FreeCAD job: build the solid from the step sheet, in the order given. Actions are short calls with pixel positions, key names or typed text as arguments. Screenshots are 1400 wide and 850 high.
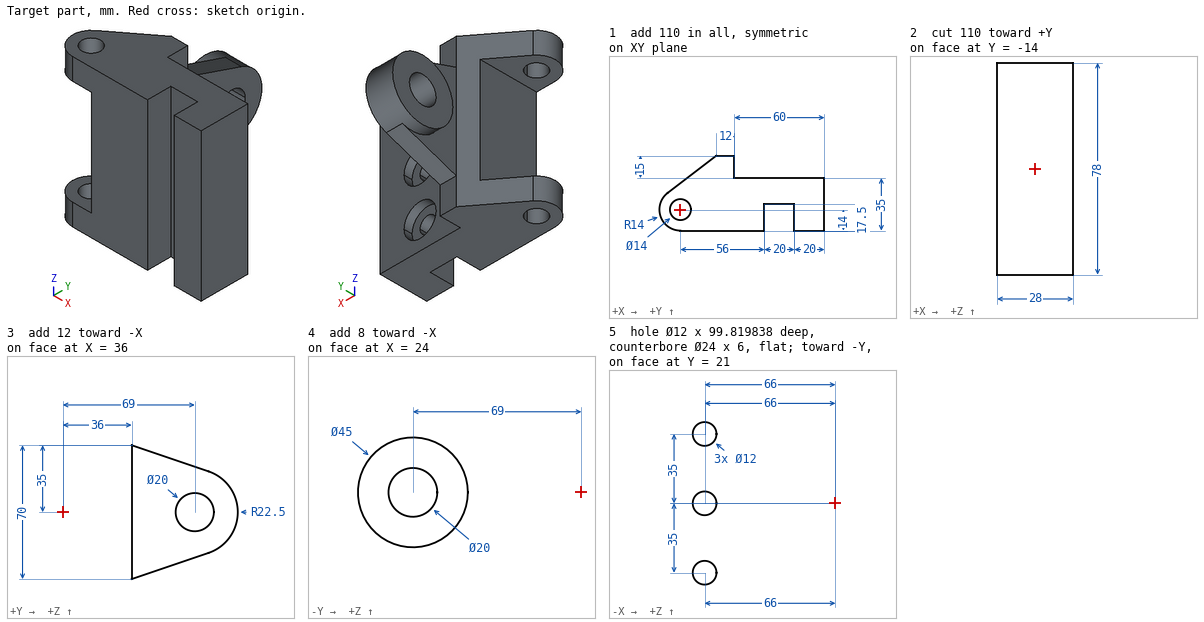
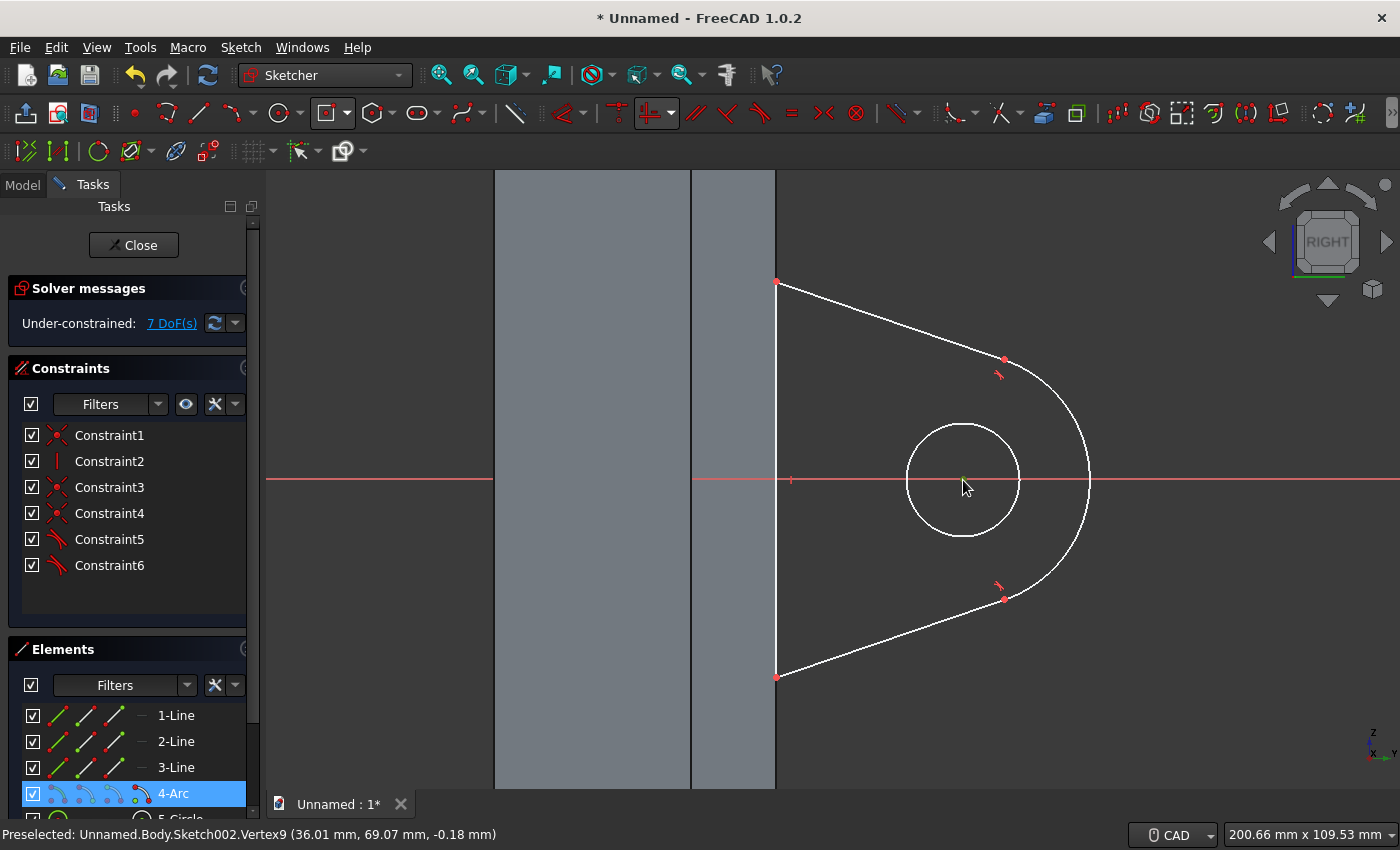
click(361, 479)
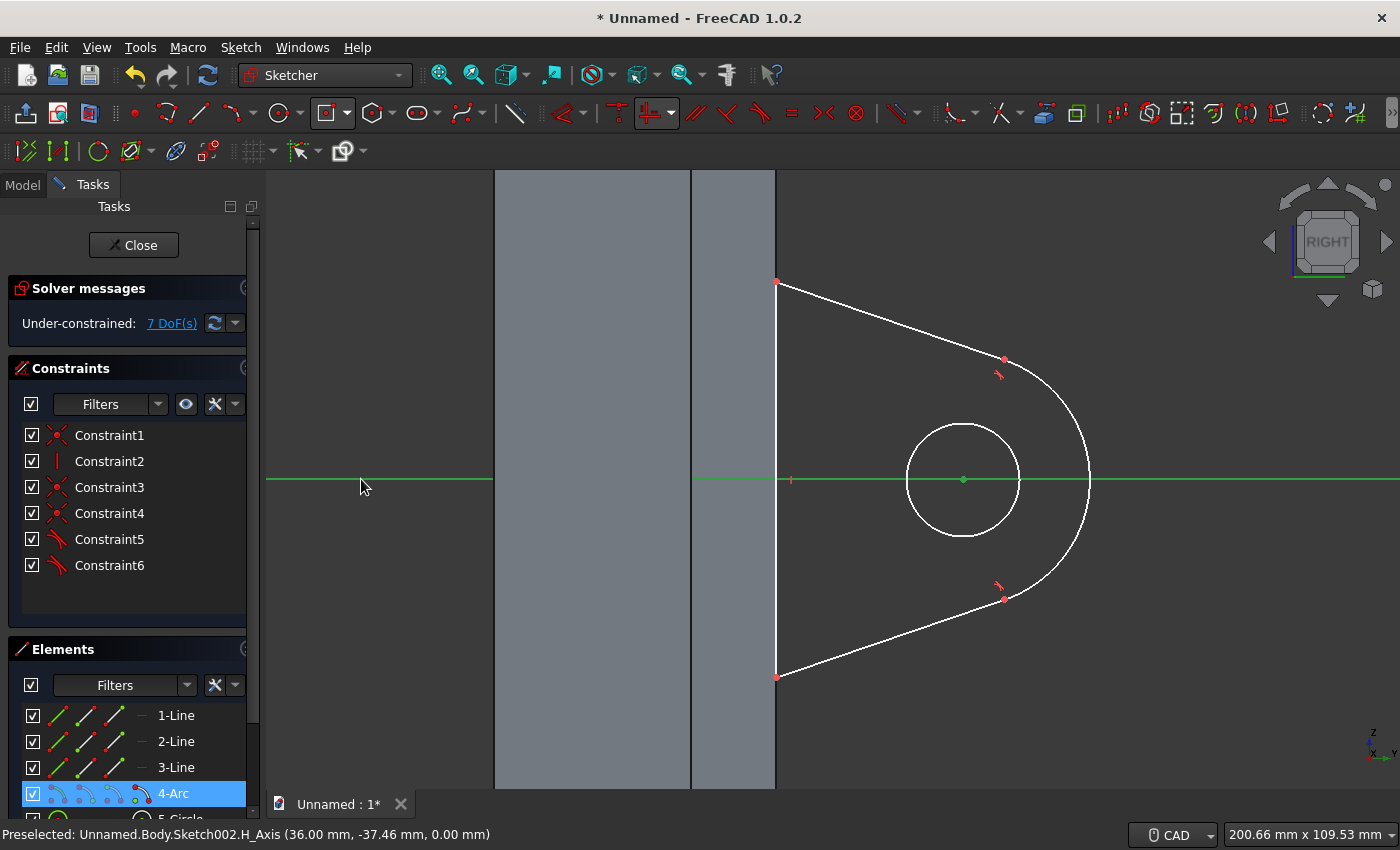
click(618, 114)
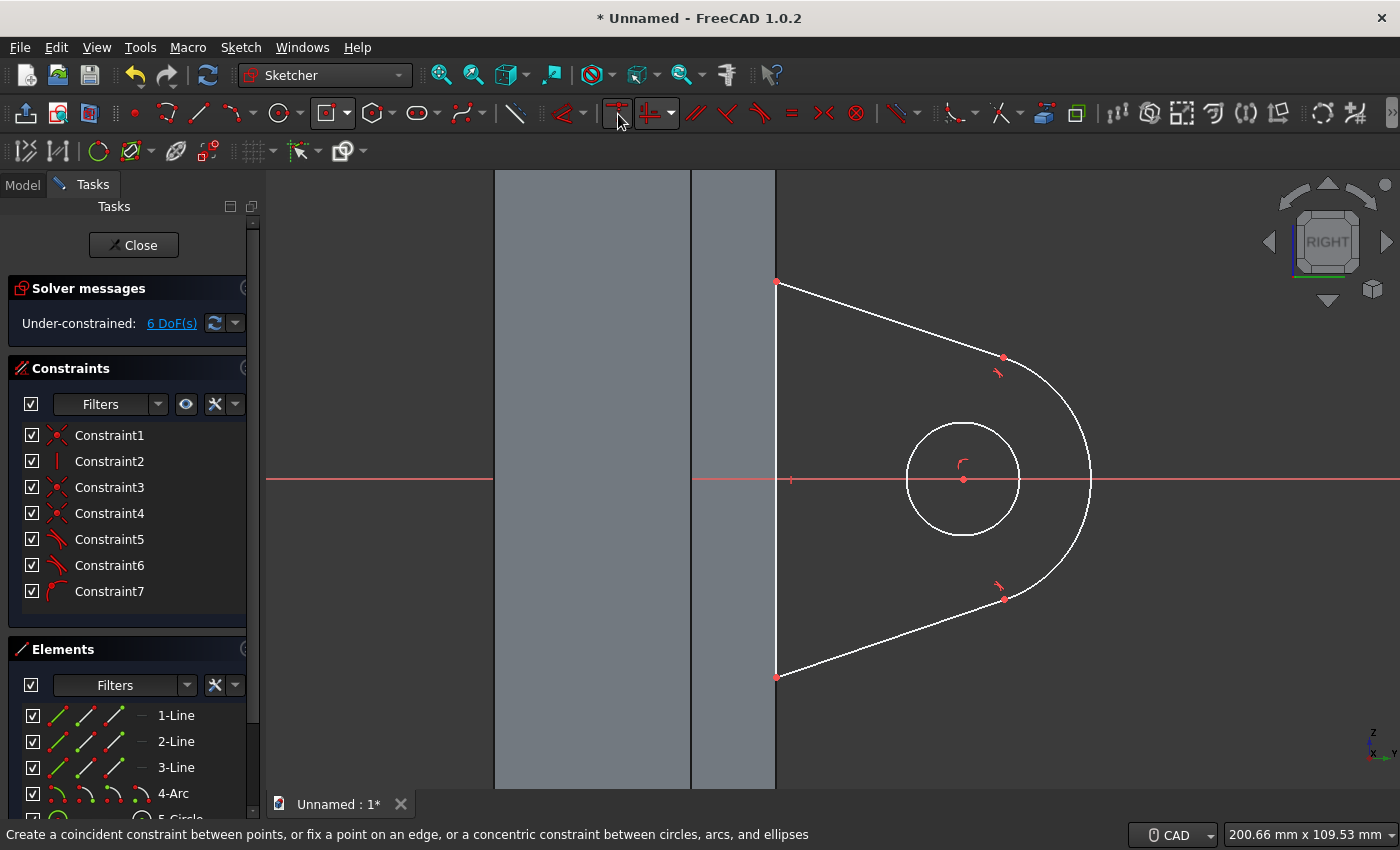
click(562, 114)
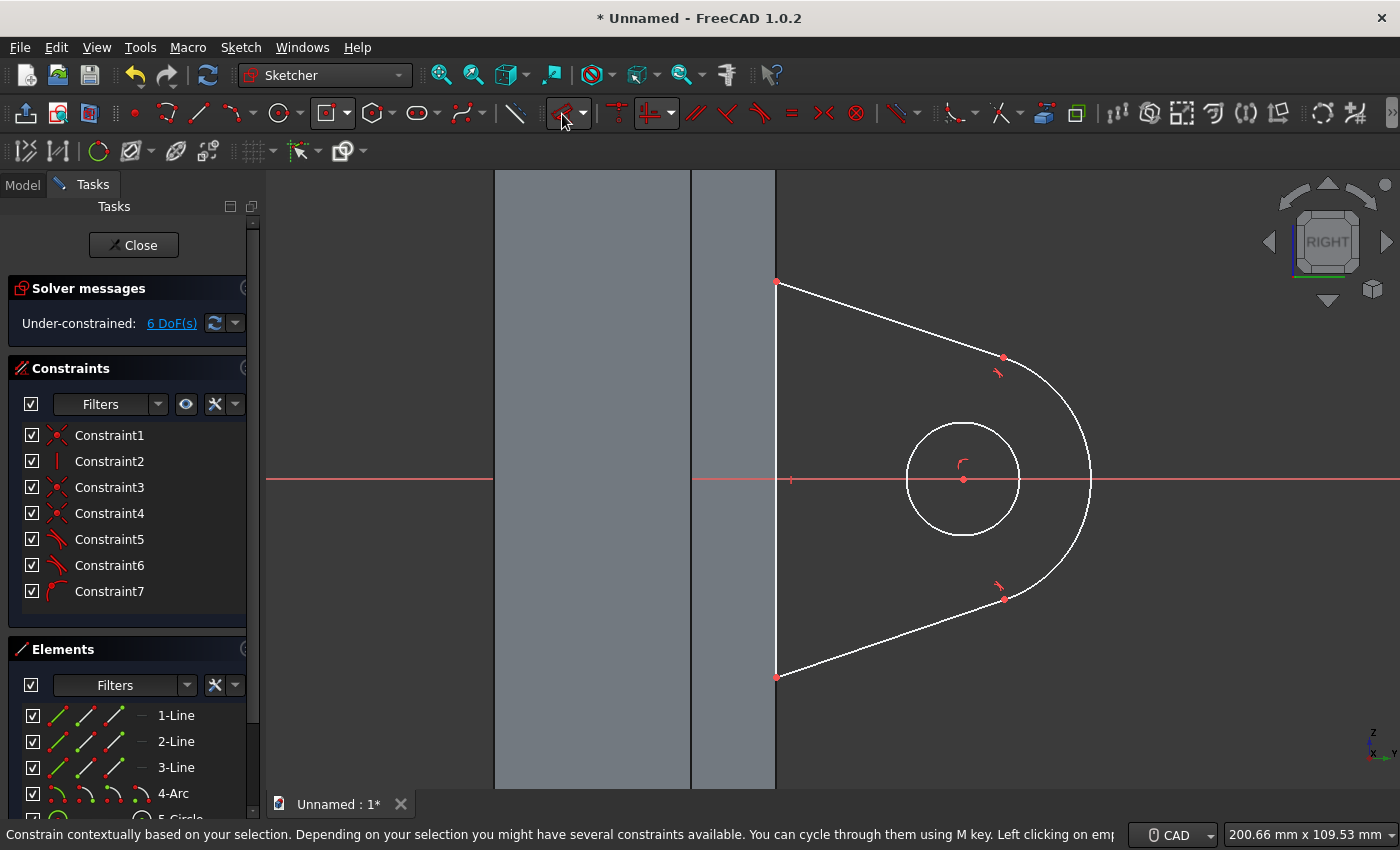
click(1076, 540)
click(1104, 555)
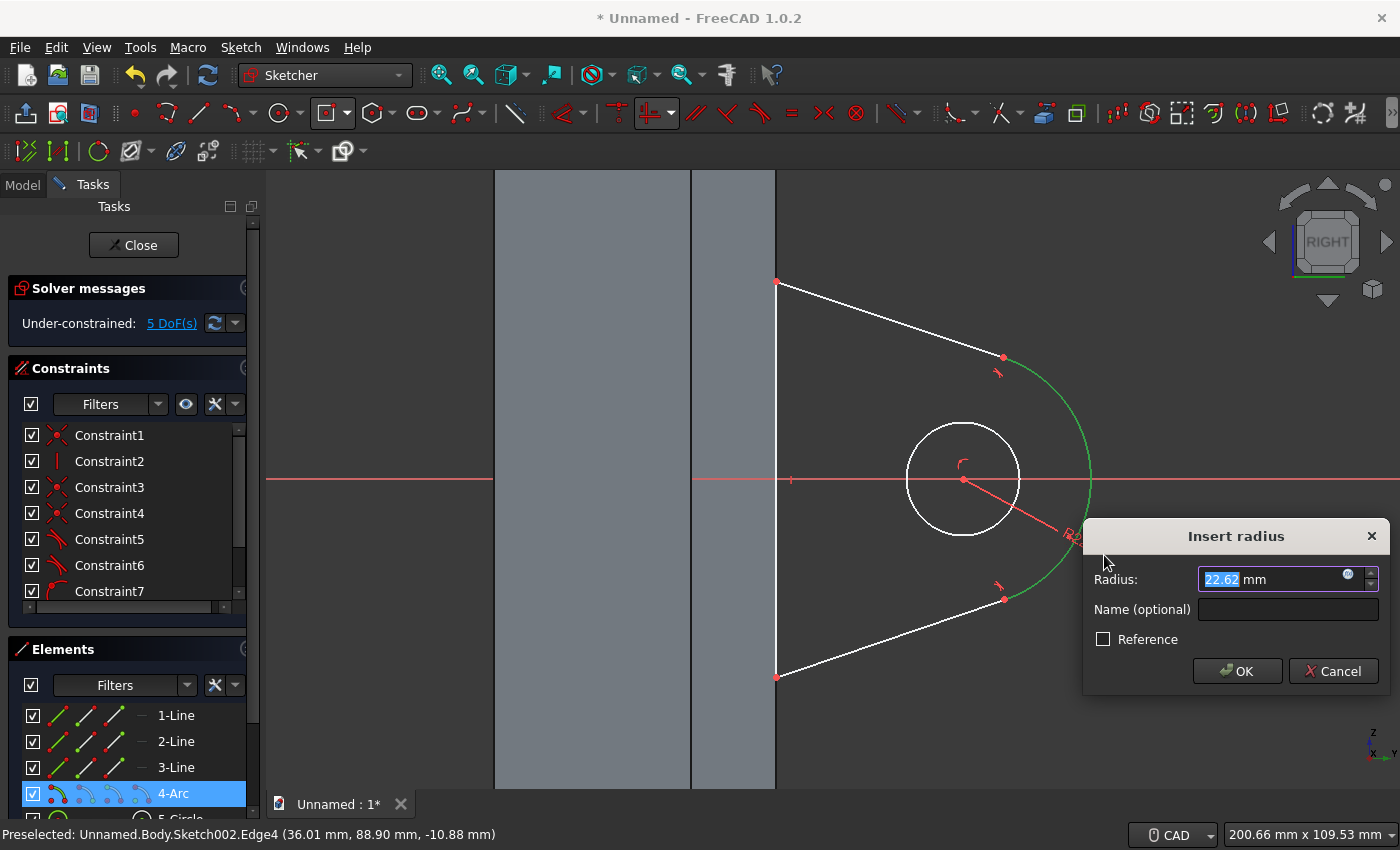
text(22.5)
key(Return)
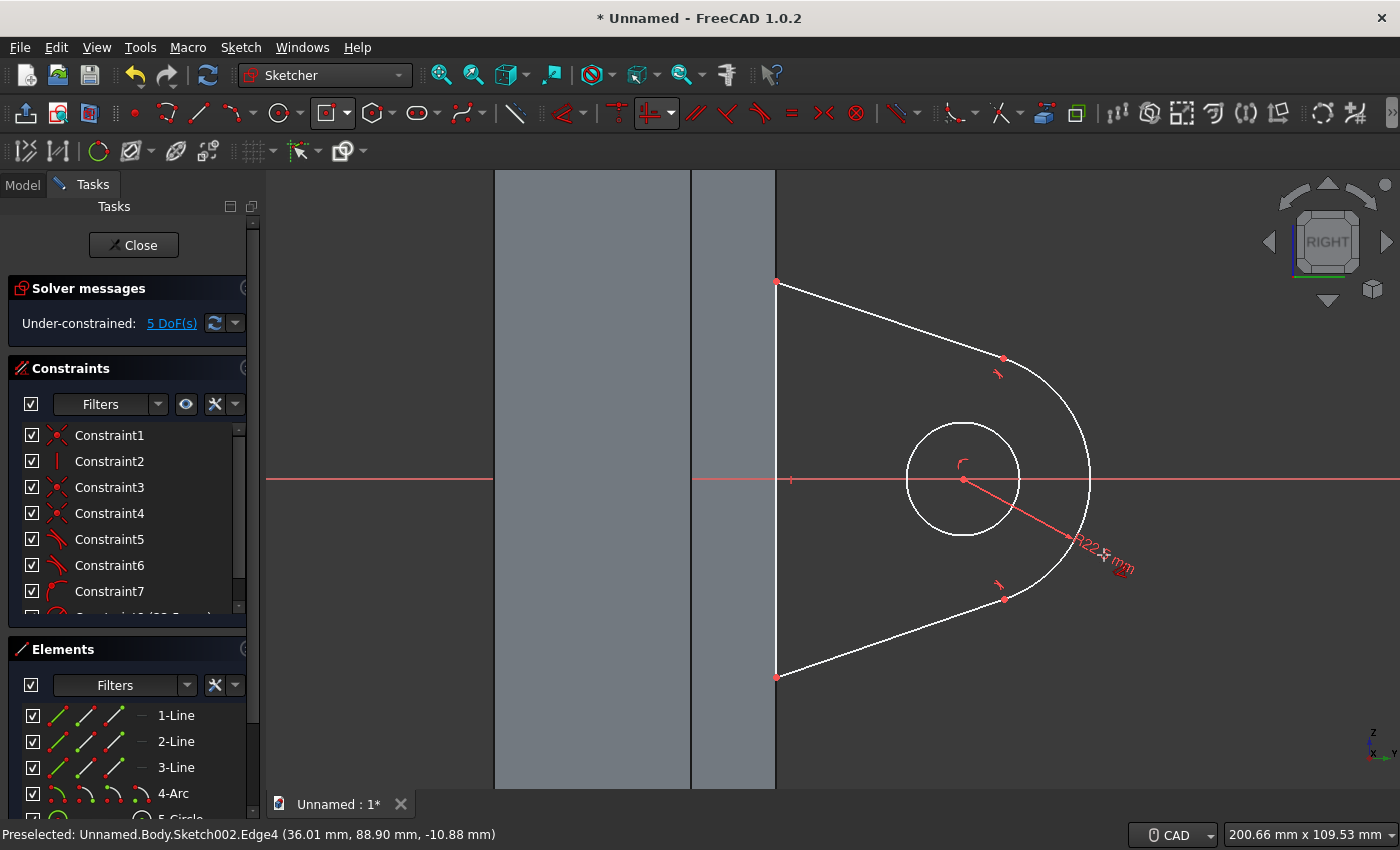
click(1003, 439)
click(1026, 416)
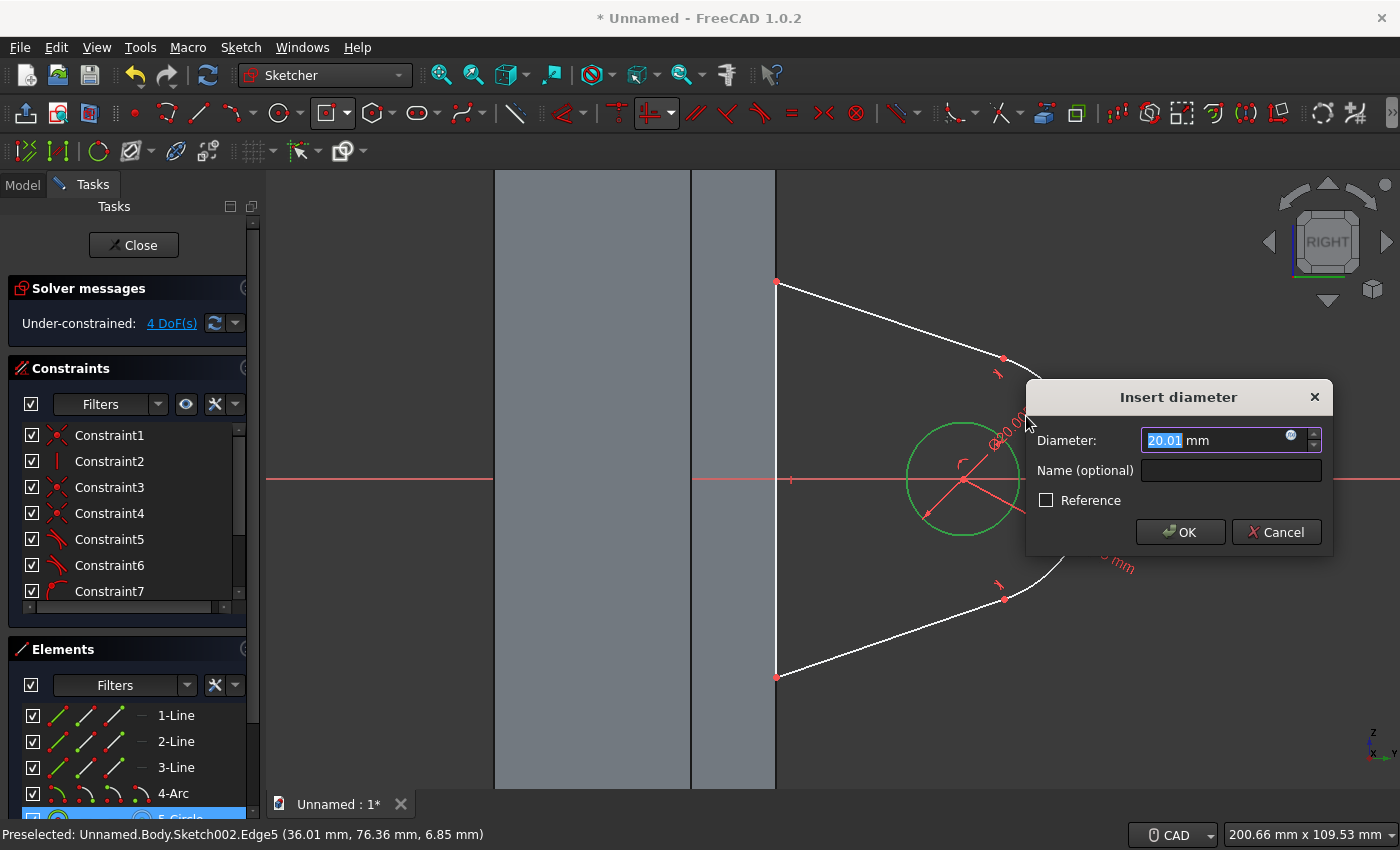
text(20)
key(Return)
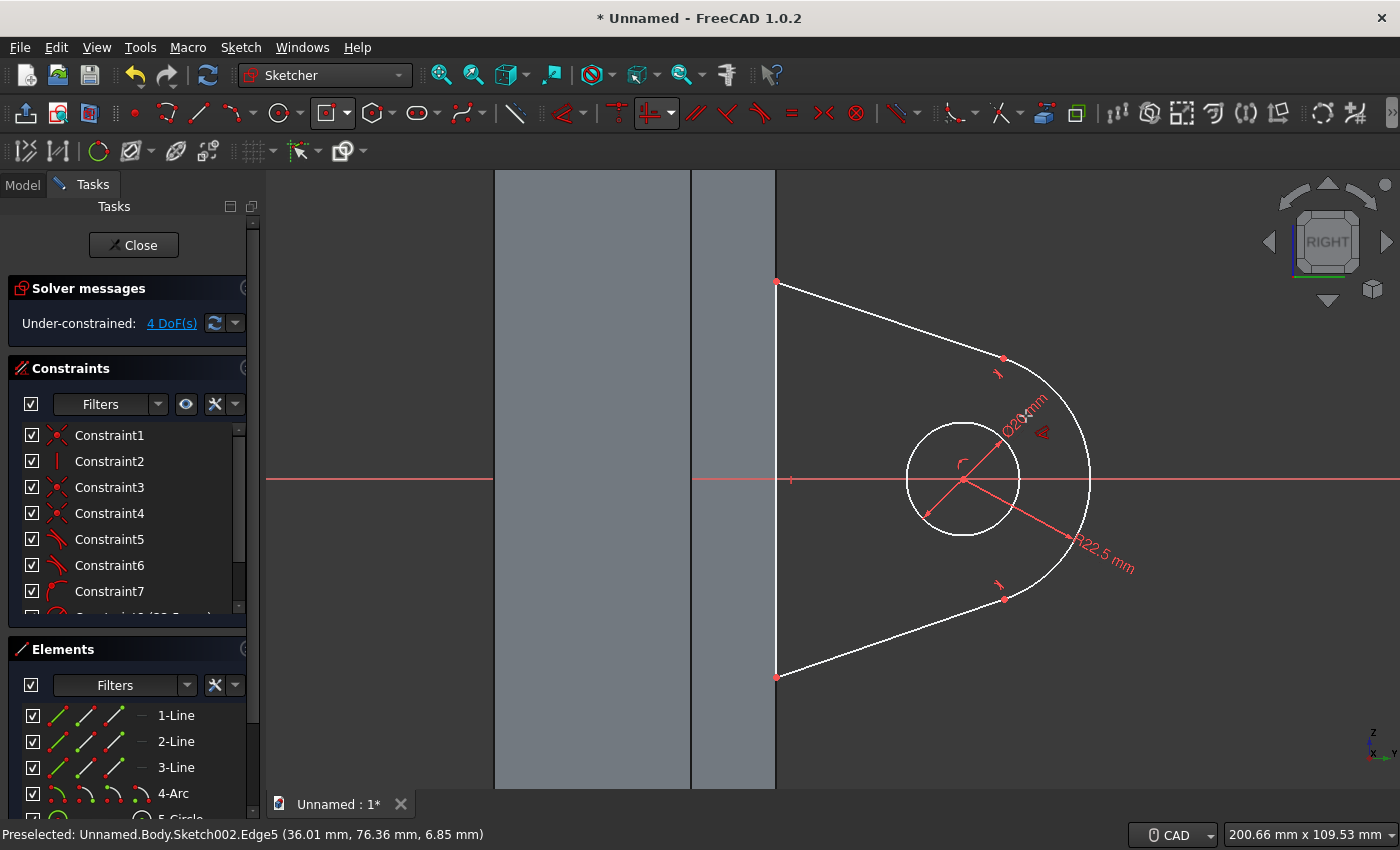
click(776, 401)
click(742, 389)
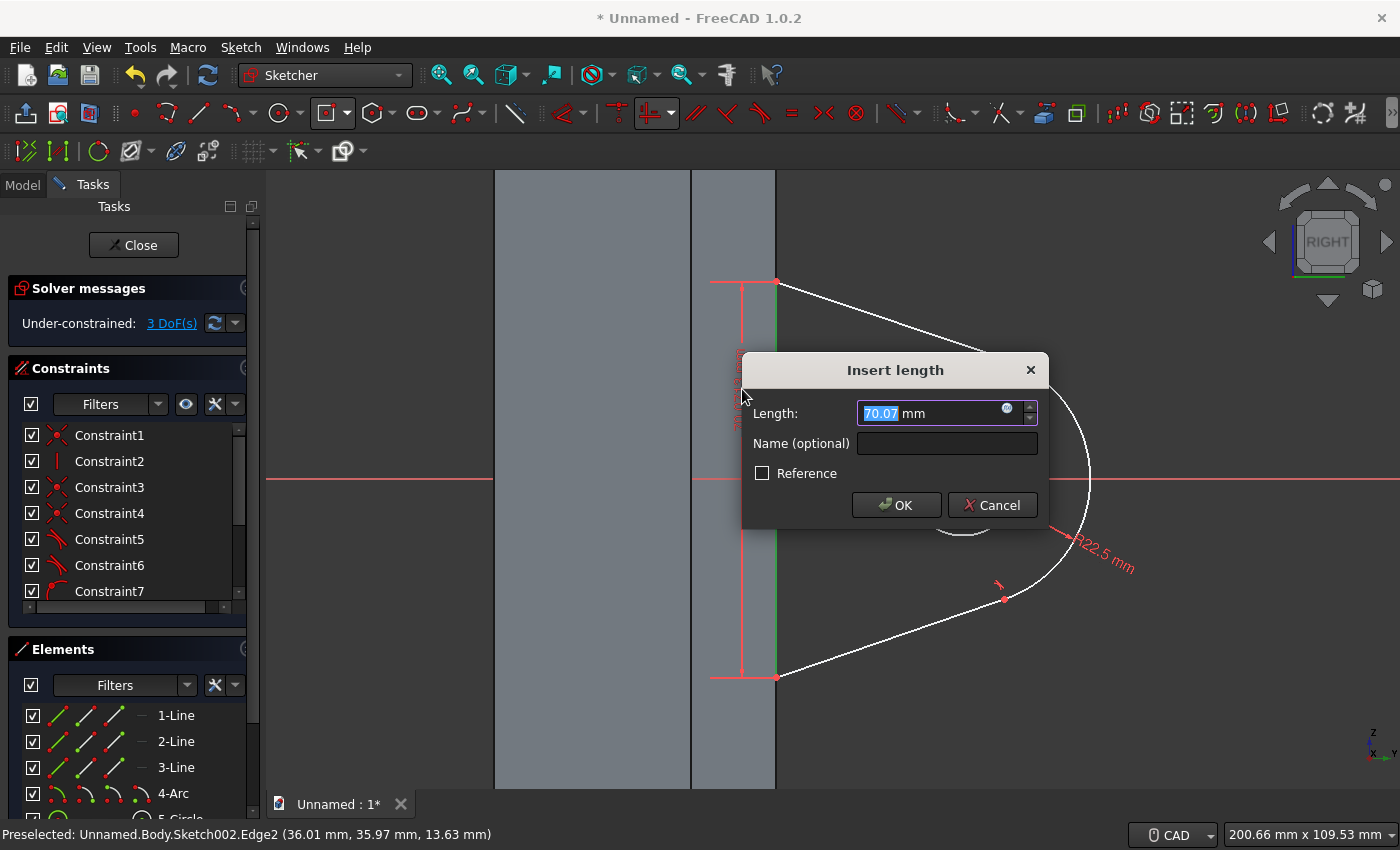
text(70)
key(Return)